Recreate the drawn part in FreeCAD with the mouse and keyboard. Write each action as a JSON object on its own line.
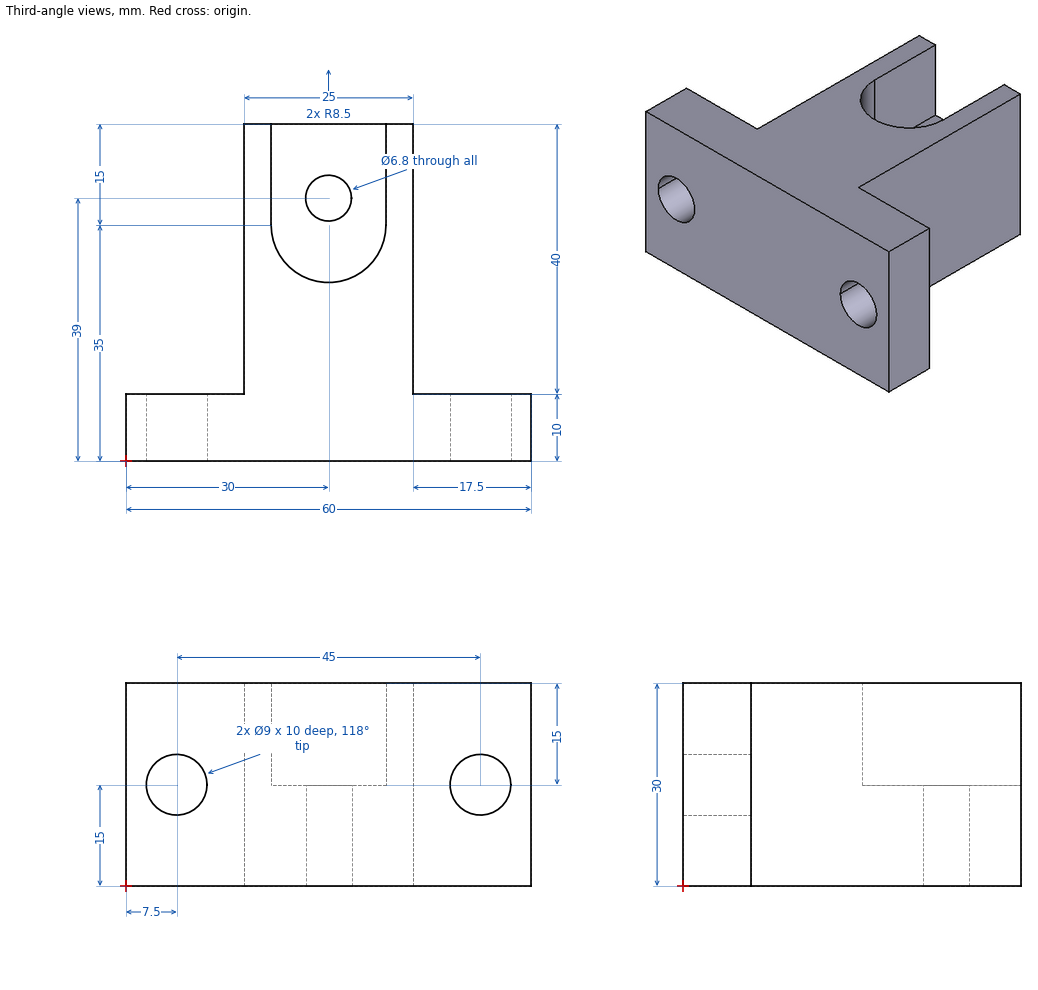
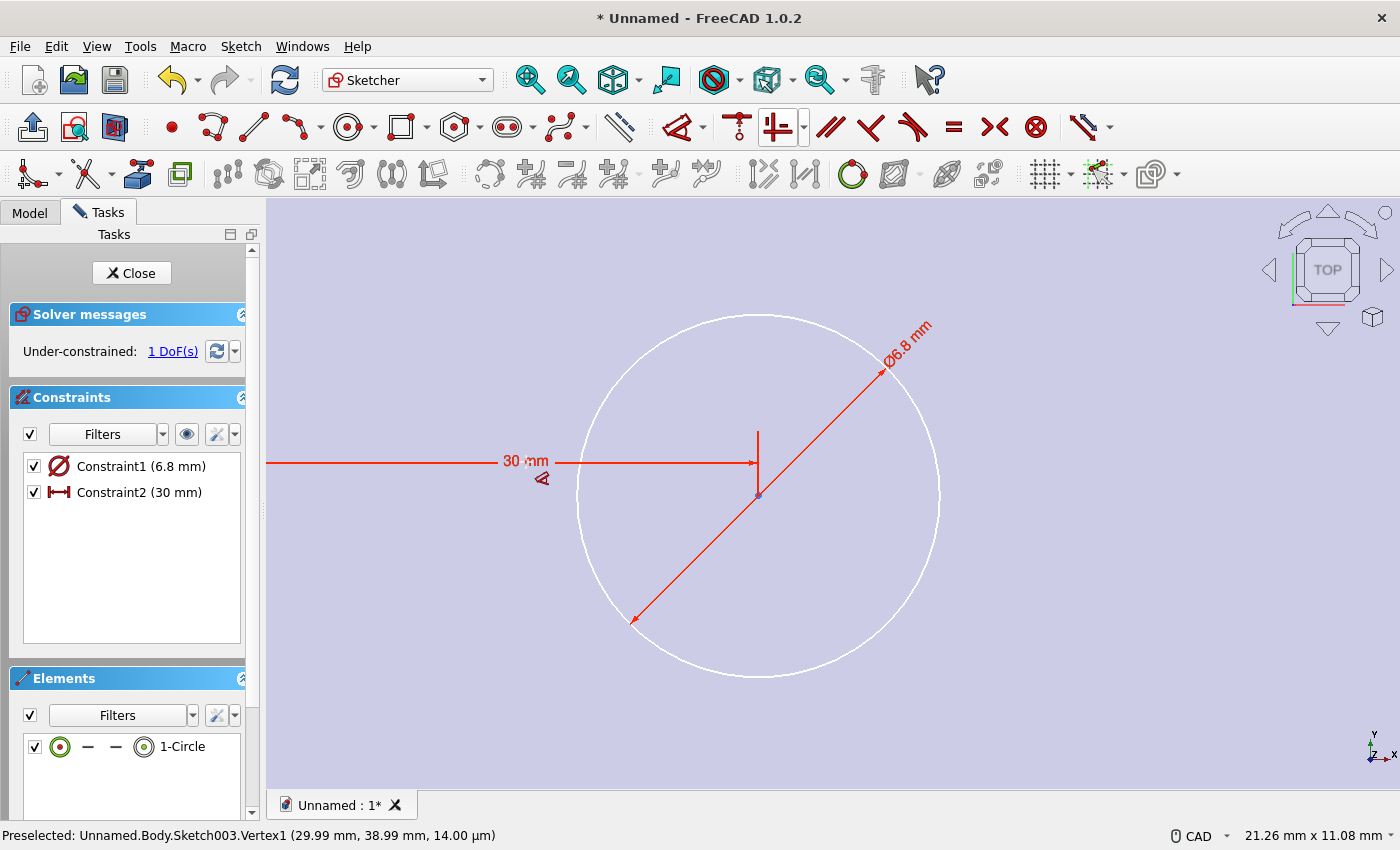
{"action": "left_click", "coordinate": [758, 496]}
{"action": "left_click", "coordinate": [792, 629]}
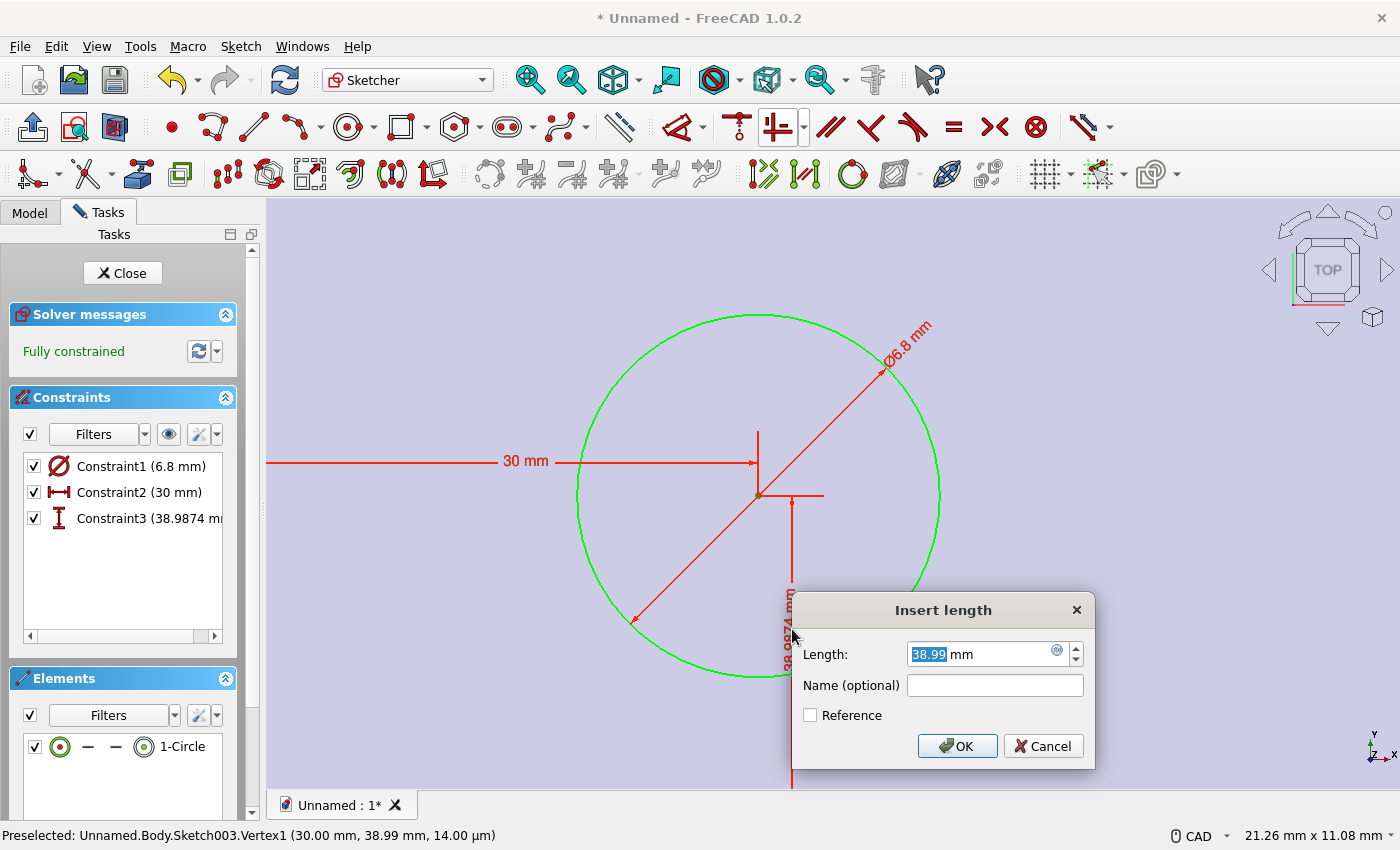
{"action": "type", "text": "39"}
{"action": "key", "text": "Return"}
{"action": "key", "text": "Escape"}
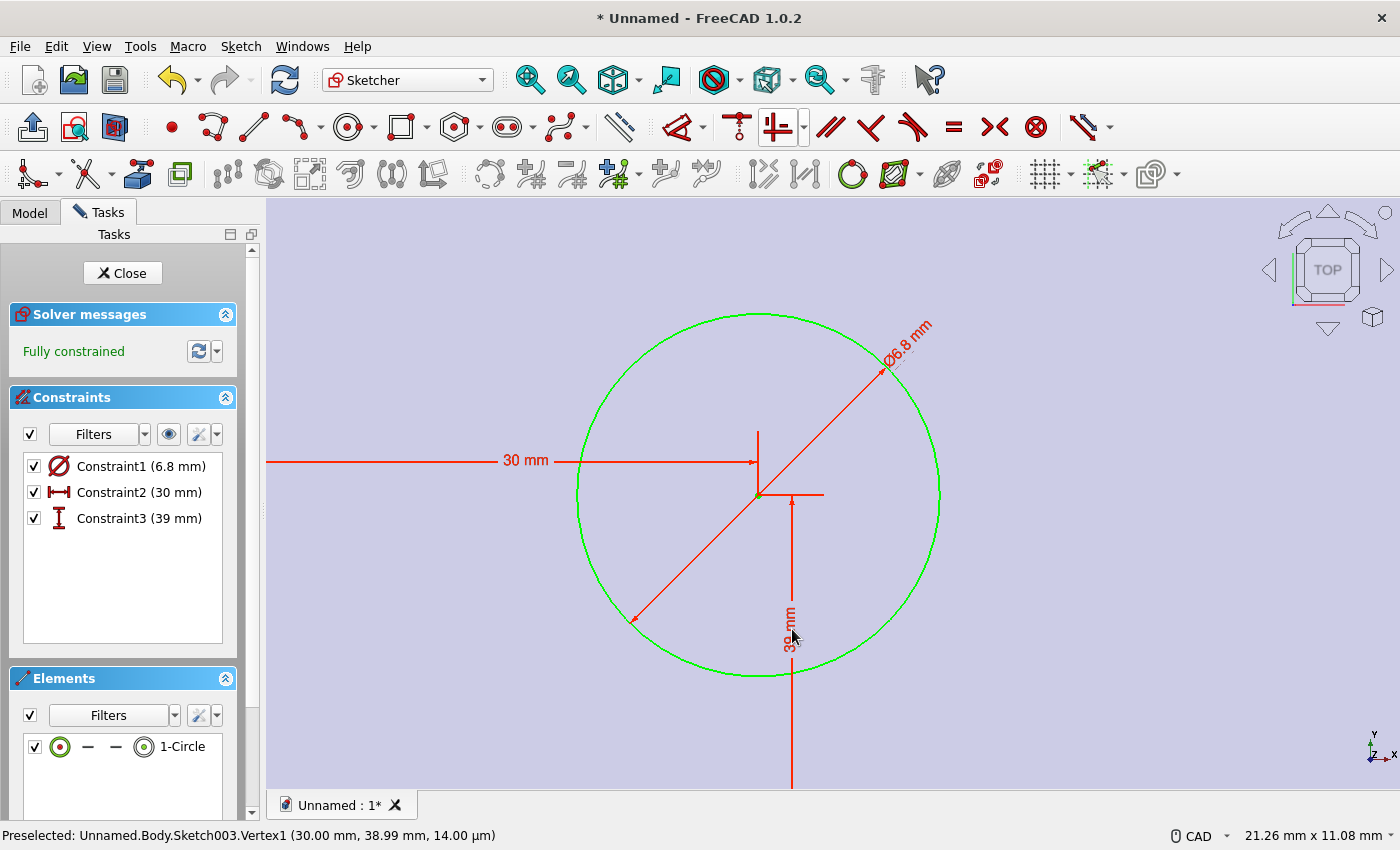
{"action": "left_click", "coordinate": [123, 273]}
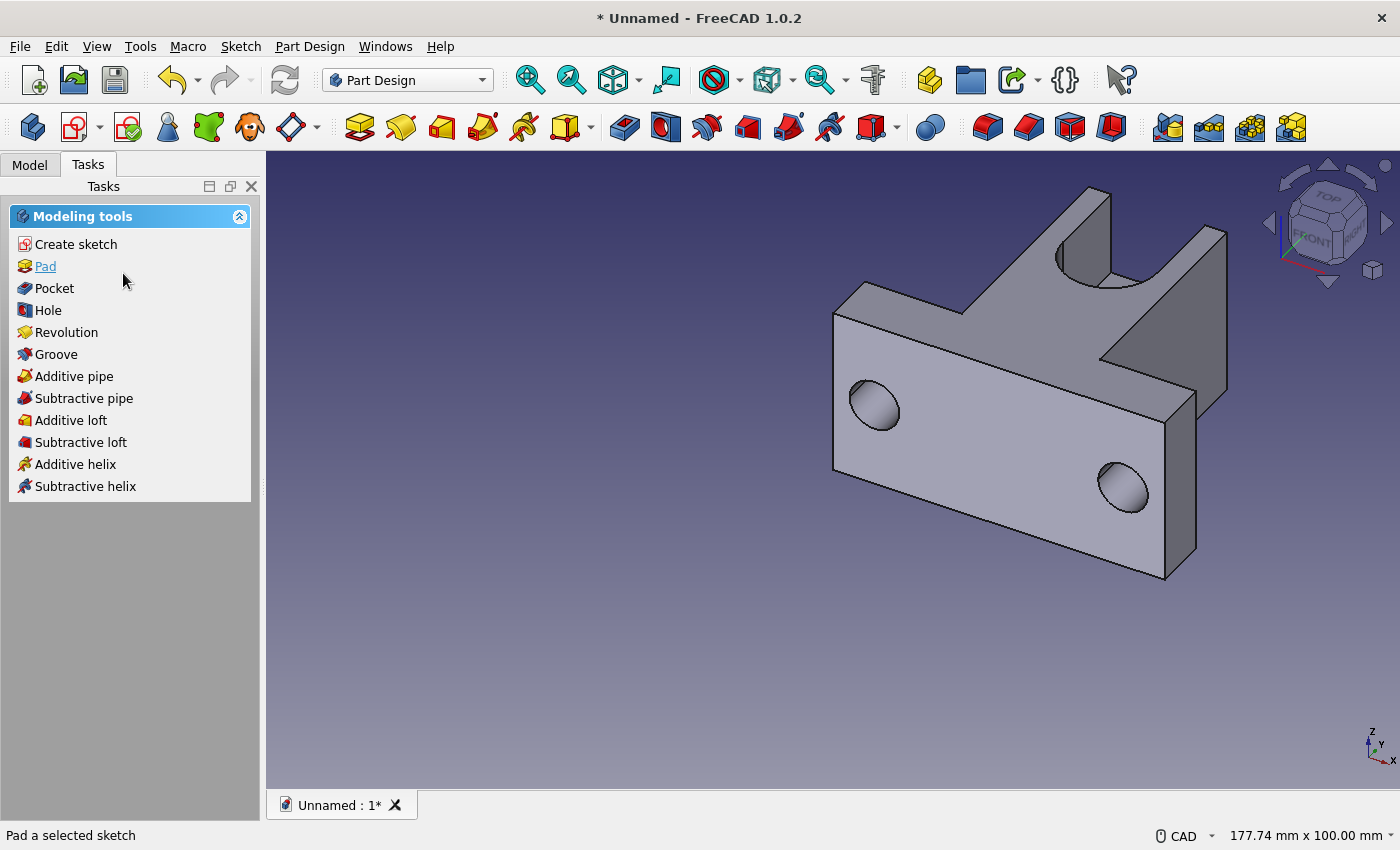
{"action": "left_click", "coordinate": [666, 128]}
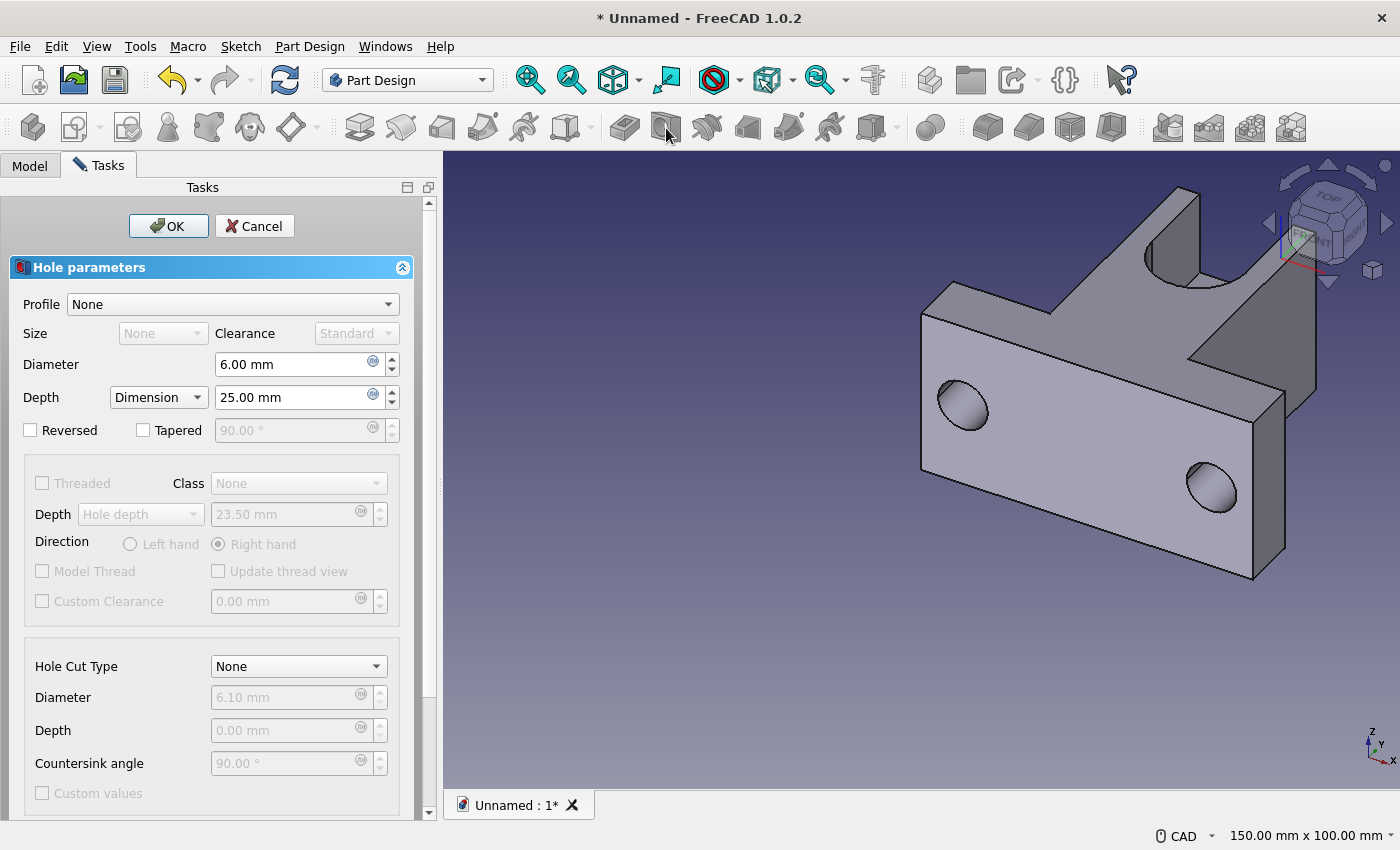
{"action": "triple_click", "coordinate": [300, 364]}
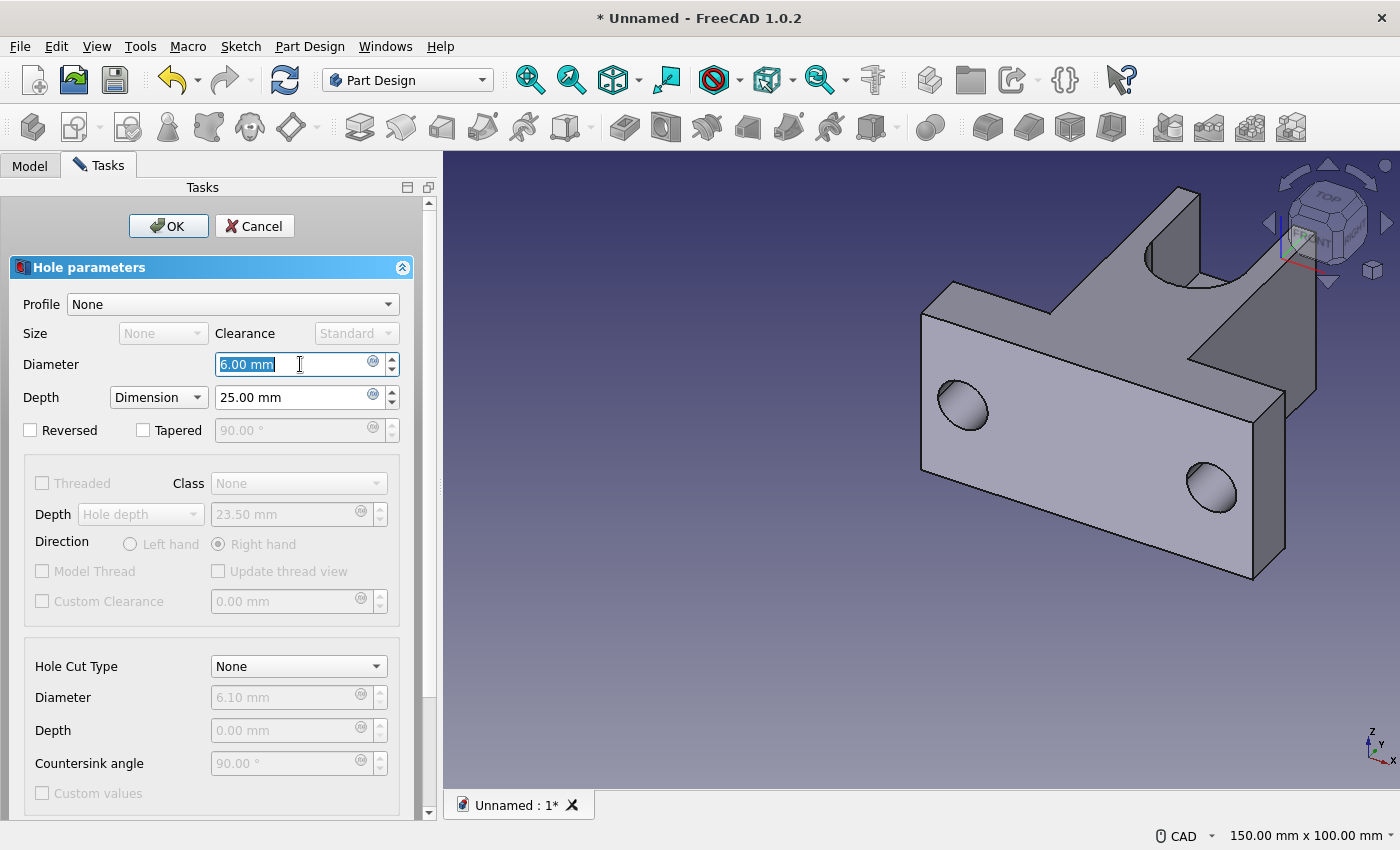
{"action": "type", "text": "6.8"}
{"action": "key", "text": "Tab"}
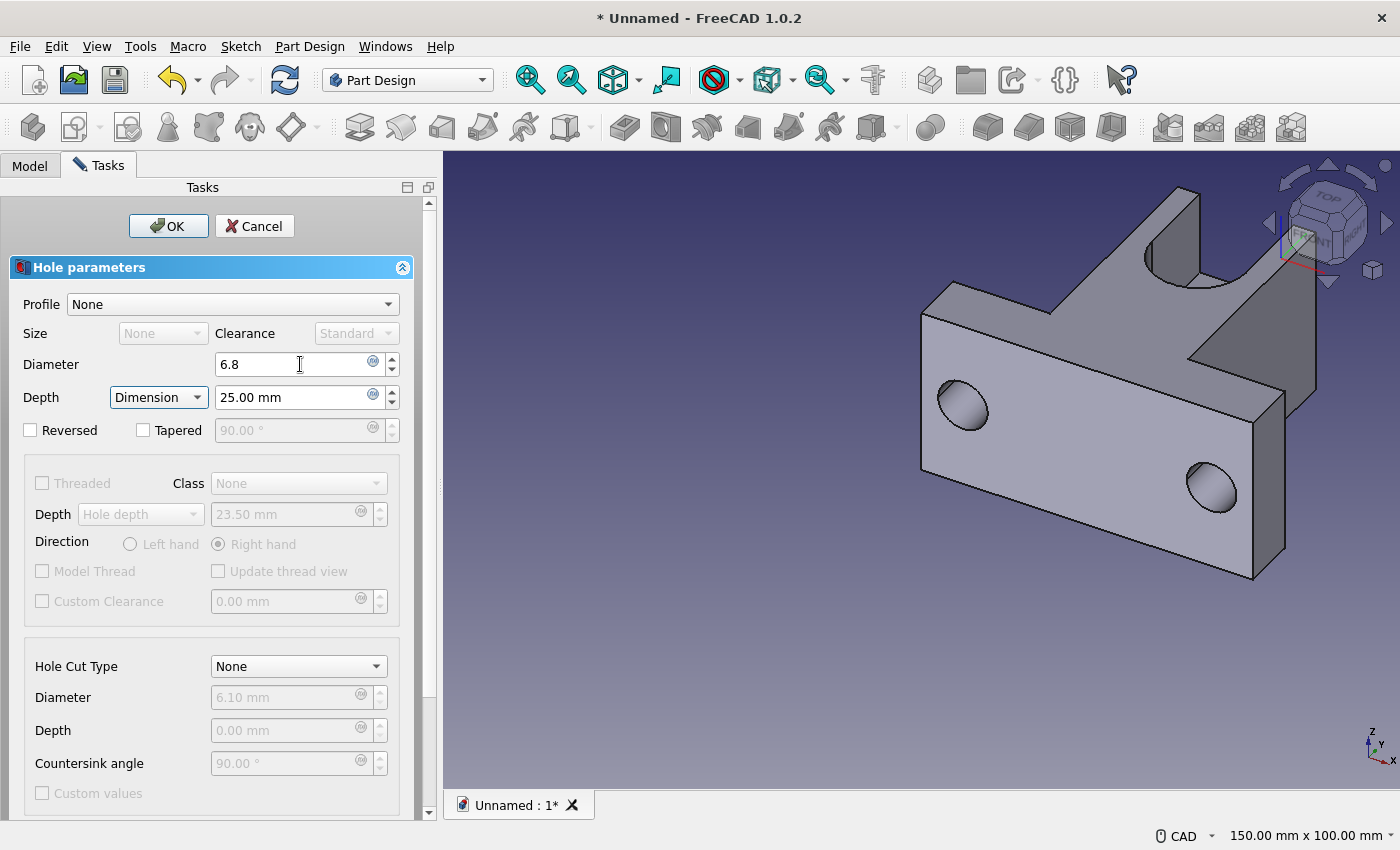
{"action": "left_click", "coordinate": [160, 398]}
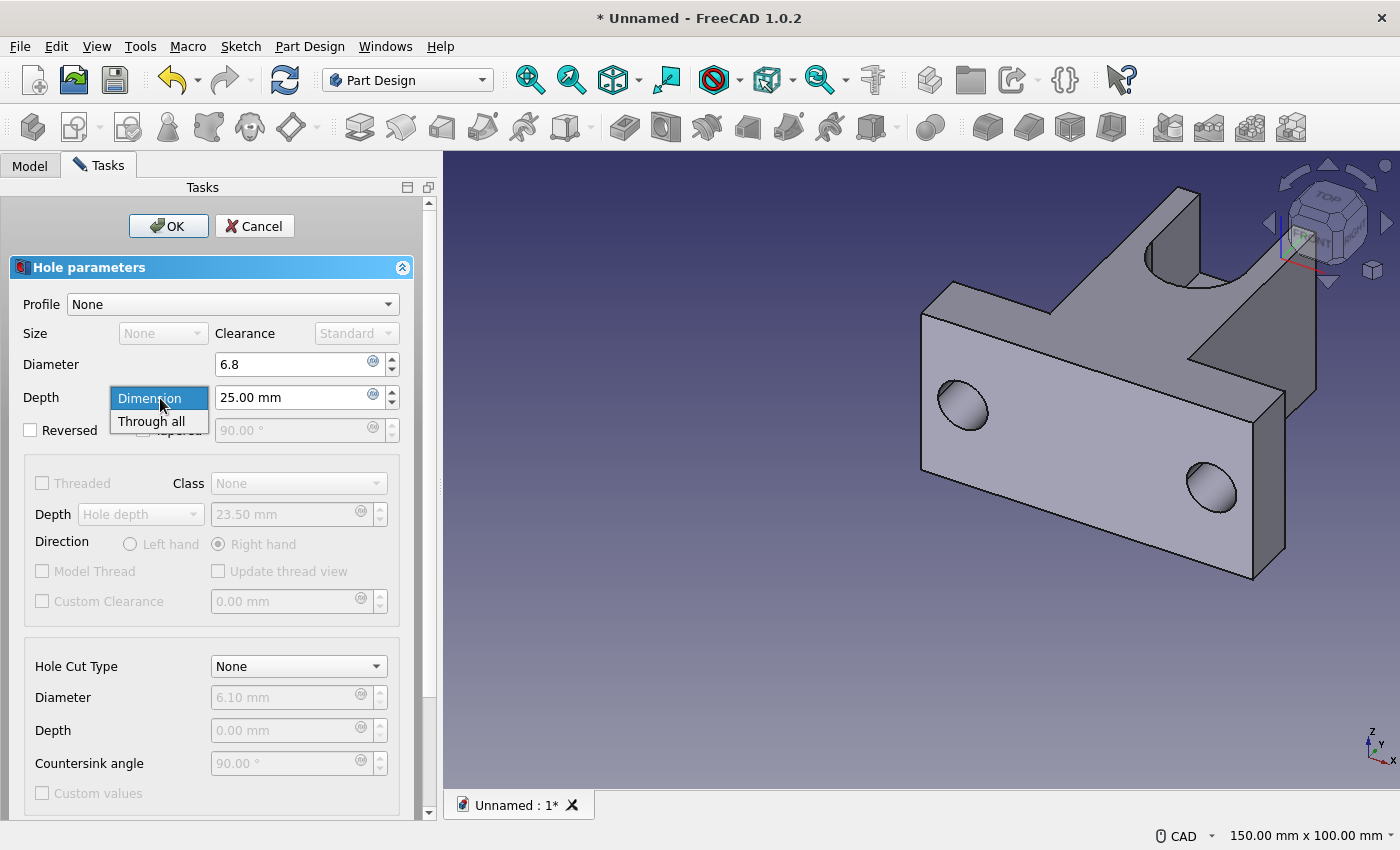
{"action": "left_click", "coordinate": [158, 422]}